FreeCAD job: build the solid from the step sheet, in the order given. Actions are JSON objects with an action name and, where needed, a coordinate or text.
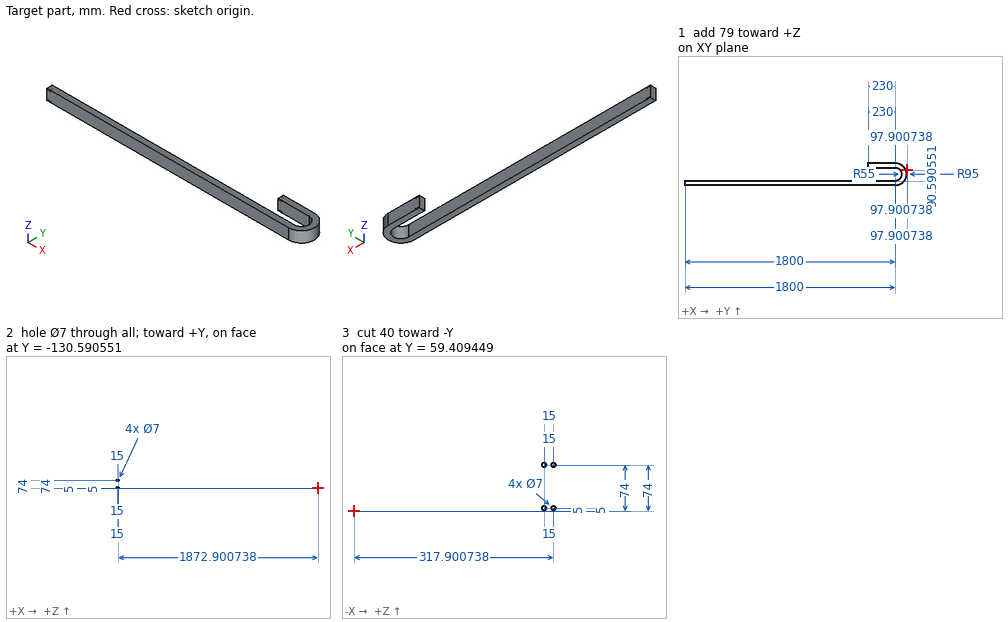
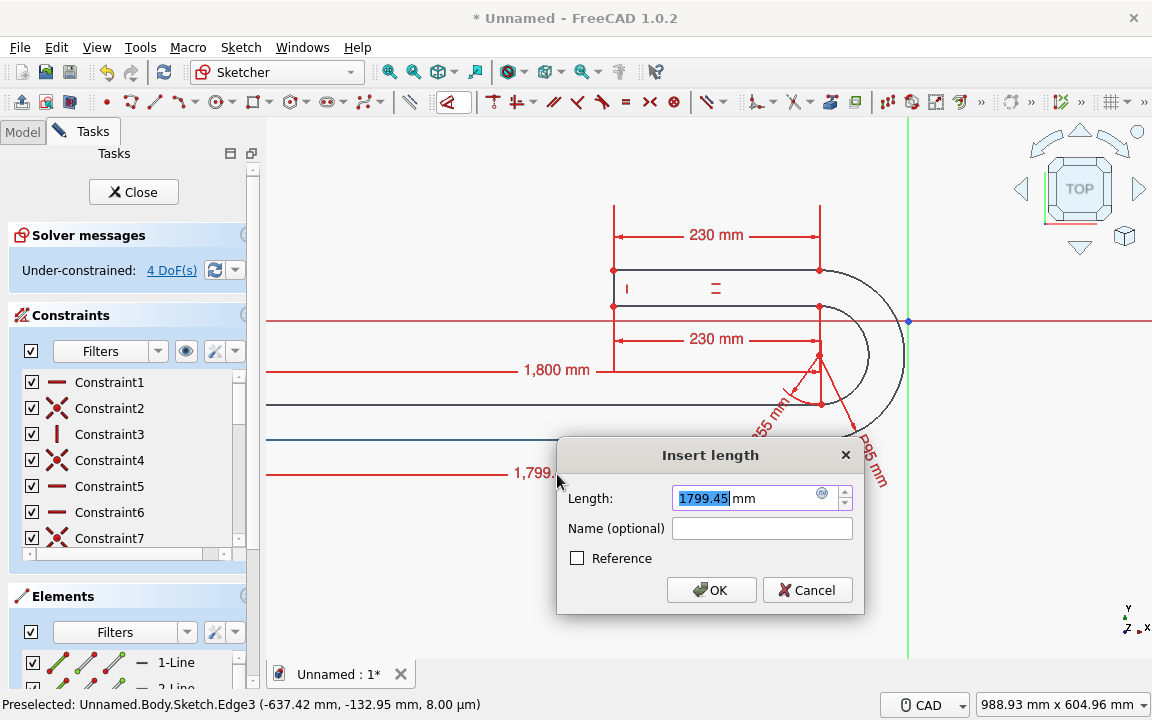
{"action": "type", "text": "1800"}
{"action": "key", "text": "Return"}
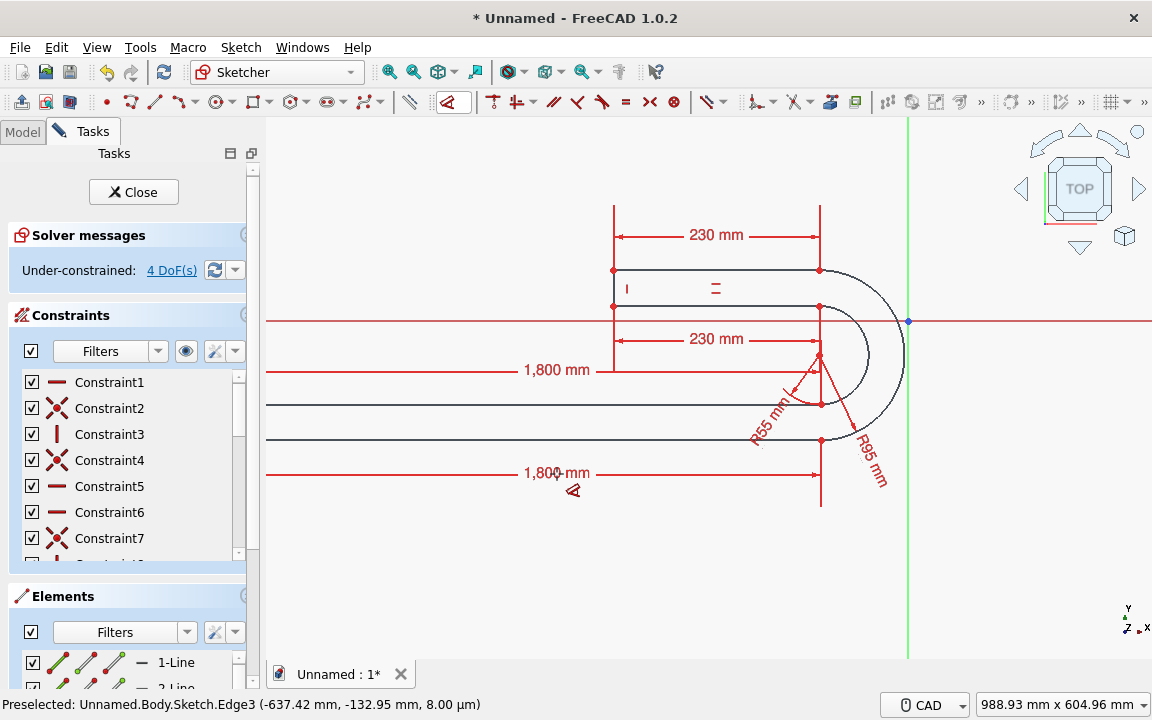
{"action": "left_click", "coordinate": [821, 405]}
{"action": "left_click", "coordinate": [885, 439]}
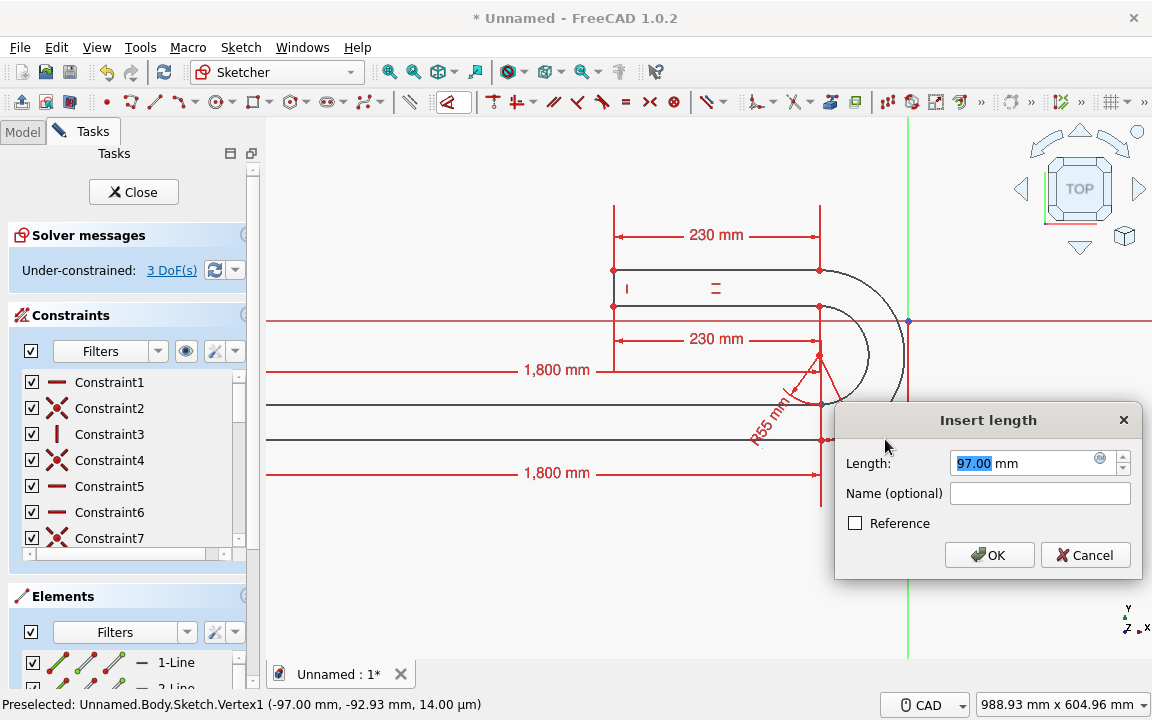
{"action": "type", "text": "97.900738"}
{"action": "key", "text": "Return"}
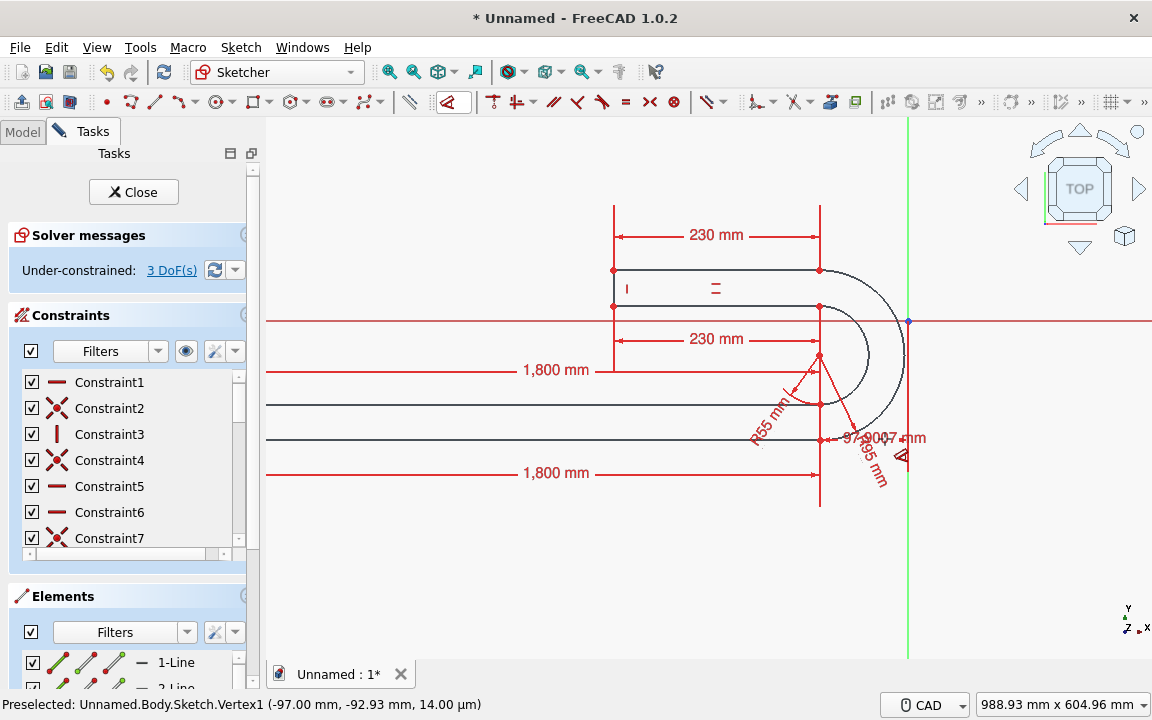
{"action": "left_click", "coordinate": [820, 405]}
{"action": "left_click", "coordinate": [942, 363]}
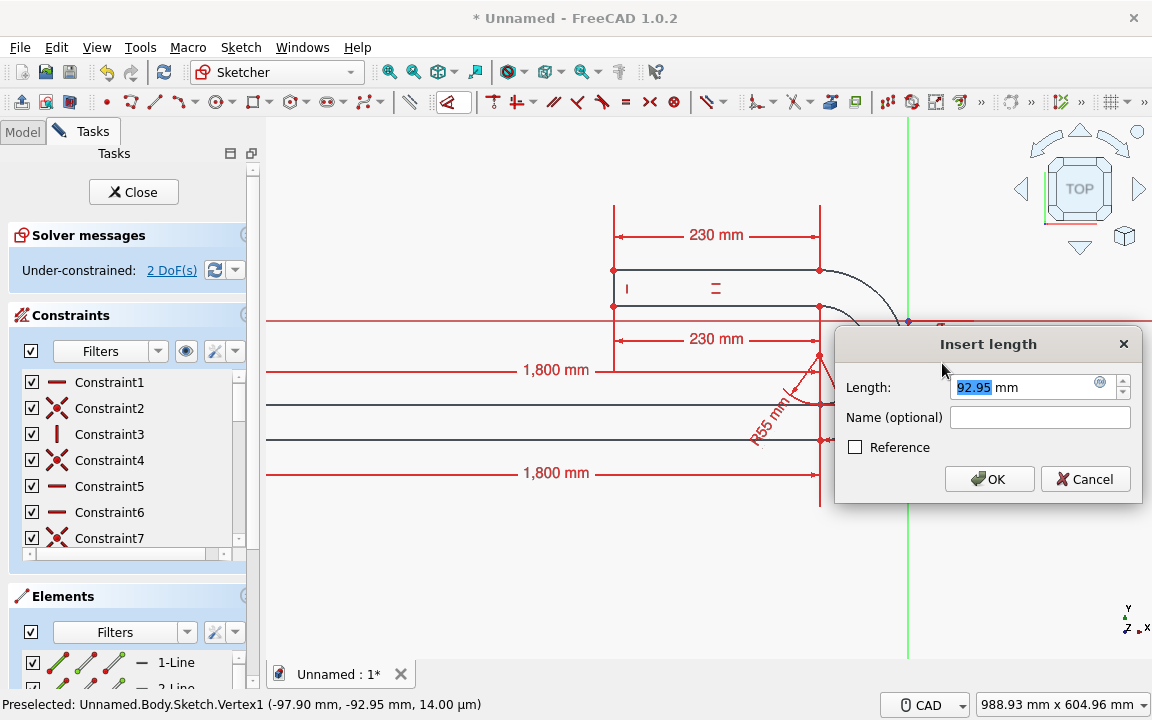
{"action": "type", "text": "90.590551"}
{"action": "key", "text": "Return"}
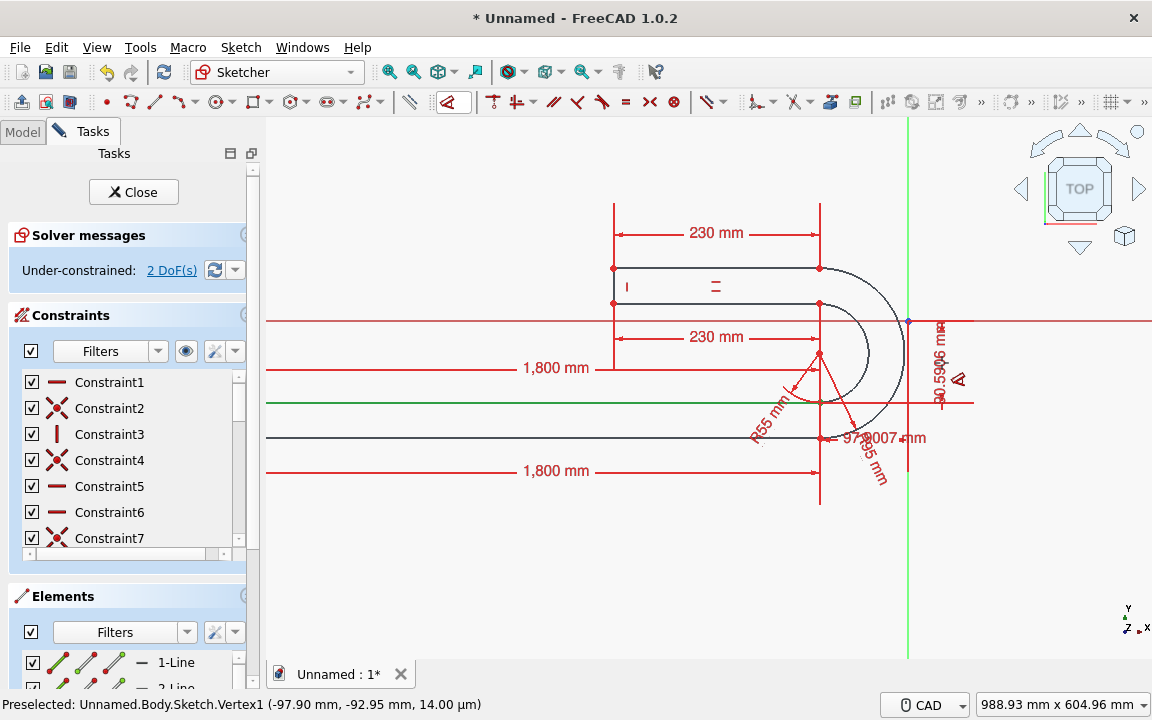
{"action": "left_click", "coordinate": [820, 268]}
{"action": "left_click", "coordinate": [864, 234]}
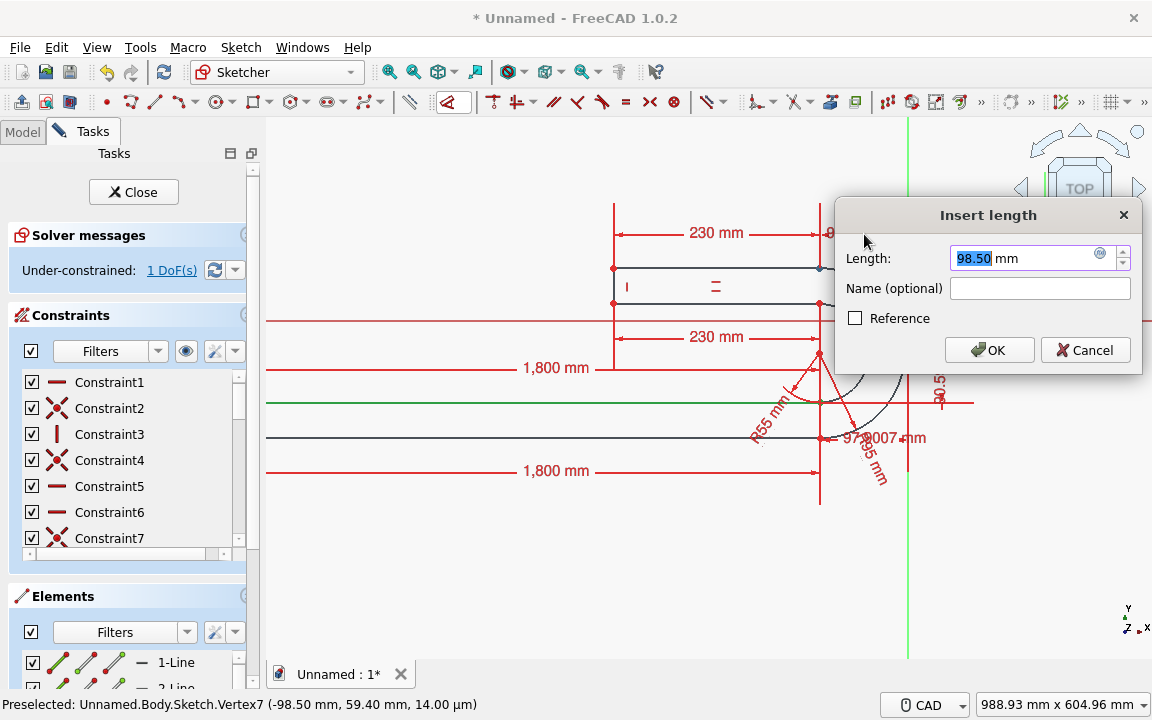
{"action": "type", "text": "97.900738"}
{"action": "key", "text": "Return"}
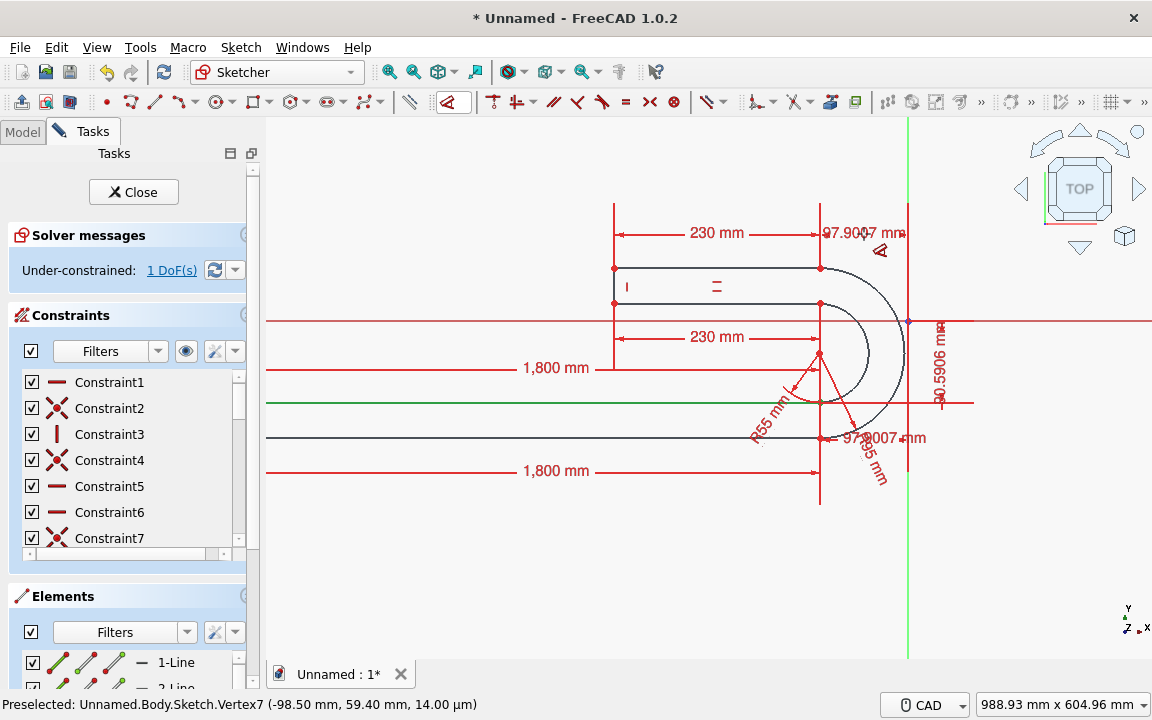
{"action": "left_click", "coordinate": [819, 353]}
{"action": "left_click", "coordinate": [843, 287]}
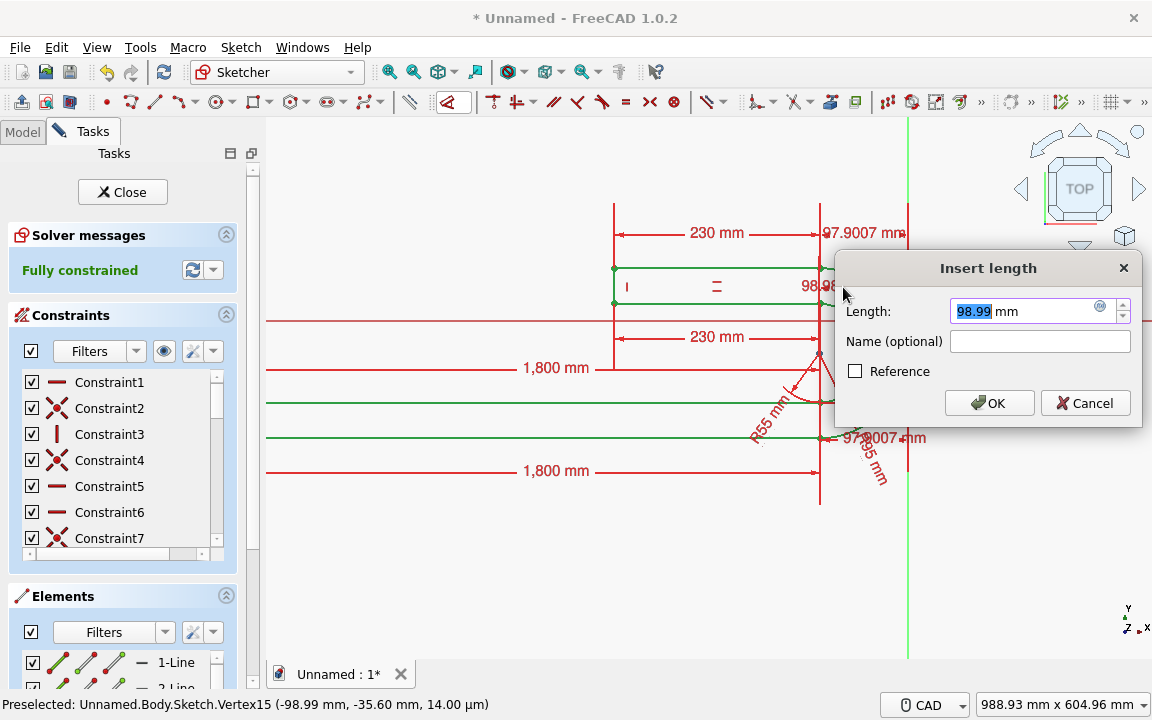
{"action": "type", "text": "97.900738"}
{"action": "key", "text": "Return"}
{"action": "key", "text": "Escape"}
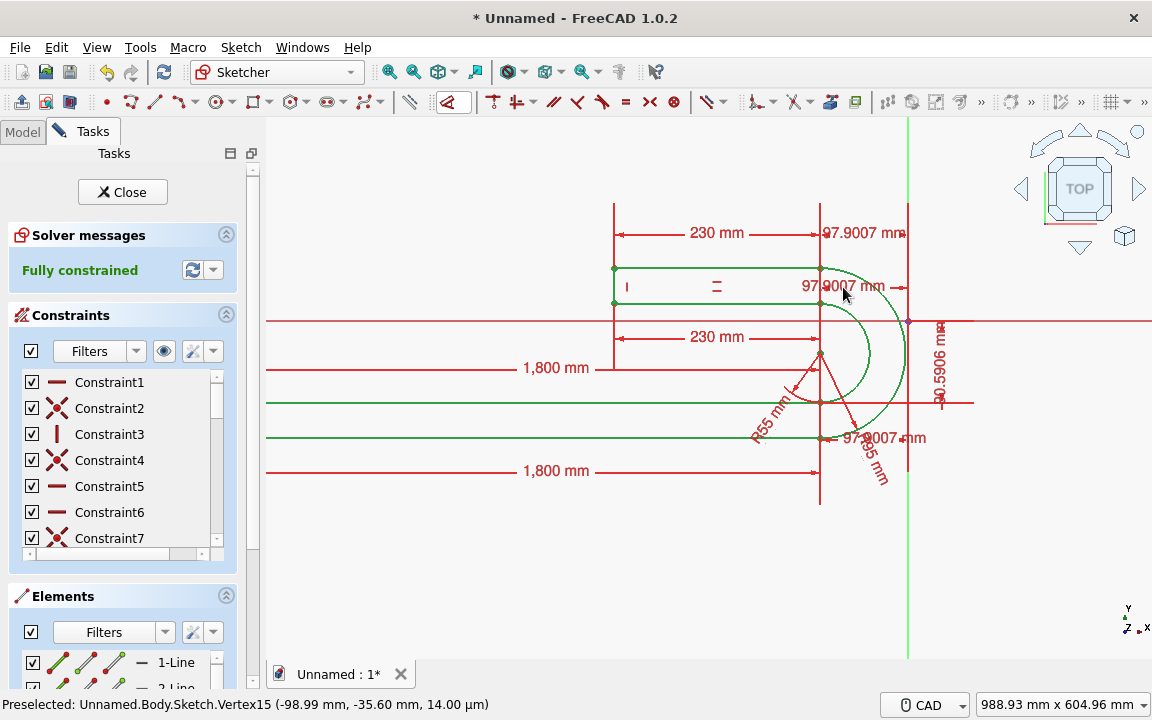
{"action": "left_click", "coordinate": [123, 192]}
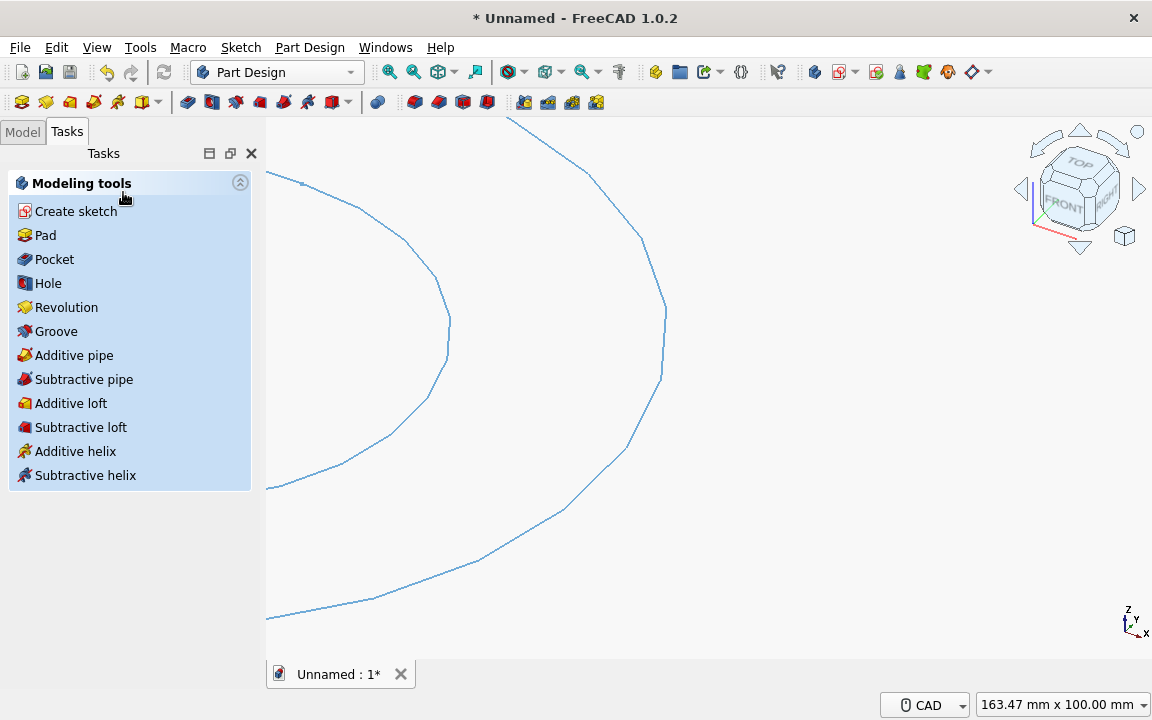
{"action": "left_click", "coordinate": [22, 102]}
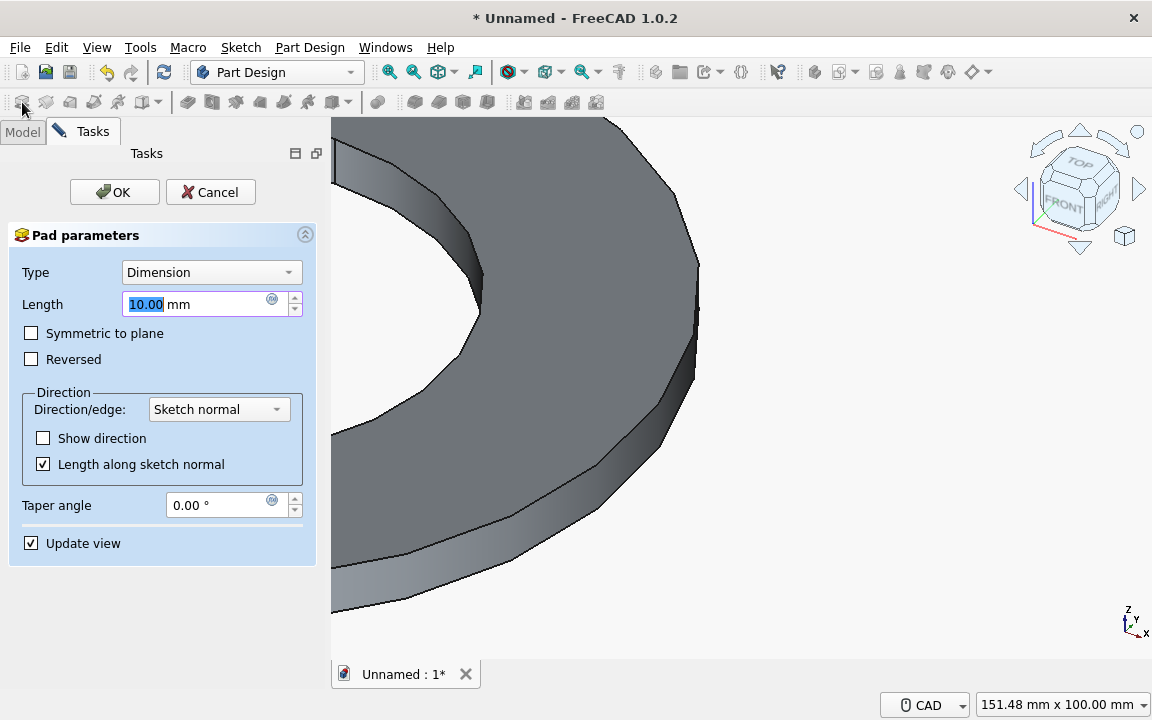
{"action": "type", "text": "79"}
{"action": "key", "text": "Tab"}